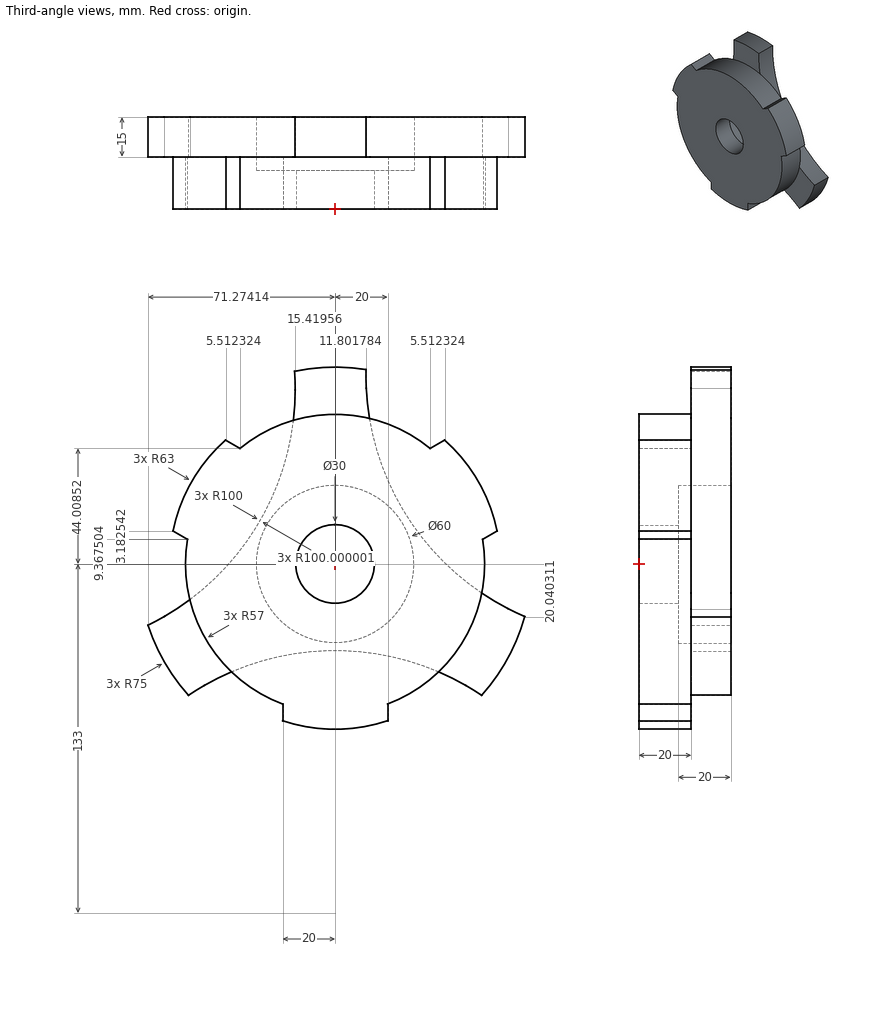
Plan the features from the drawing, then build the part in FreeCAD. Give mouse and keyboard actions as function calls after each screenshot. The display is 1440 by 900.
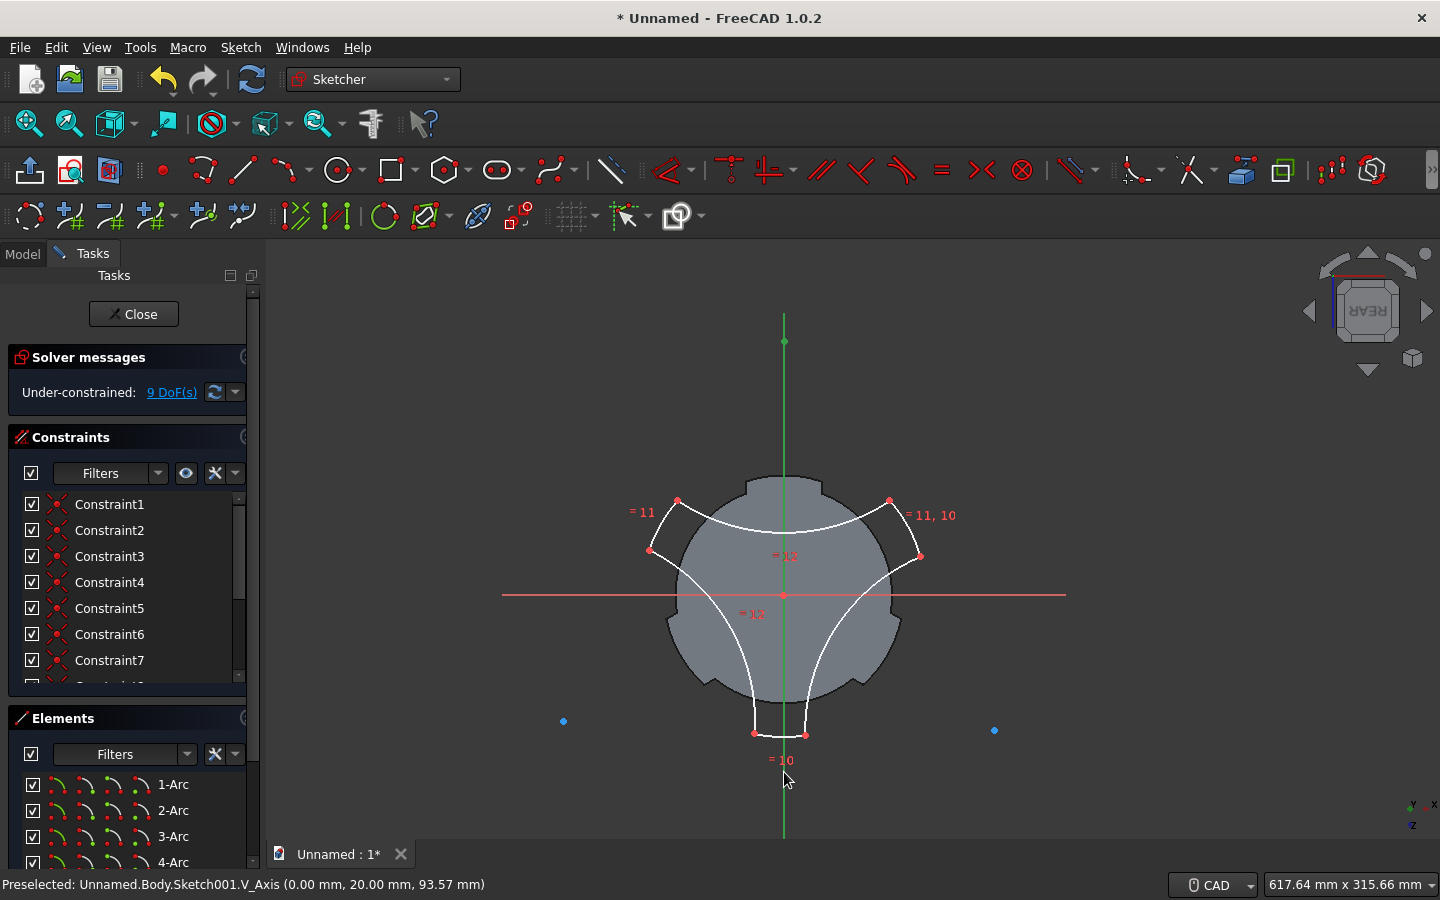
click(730, 170)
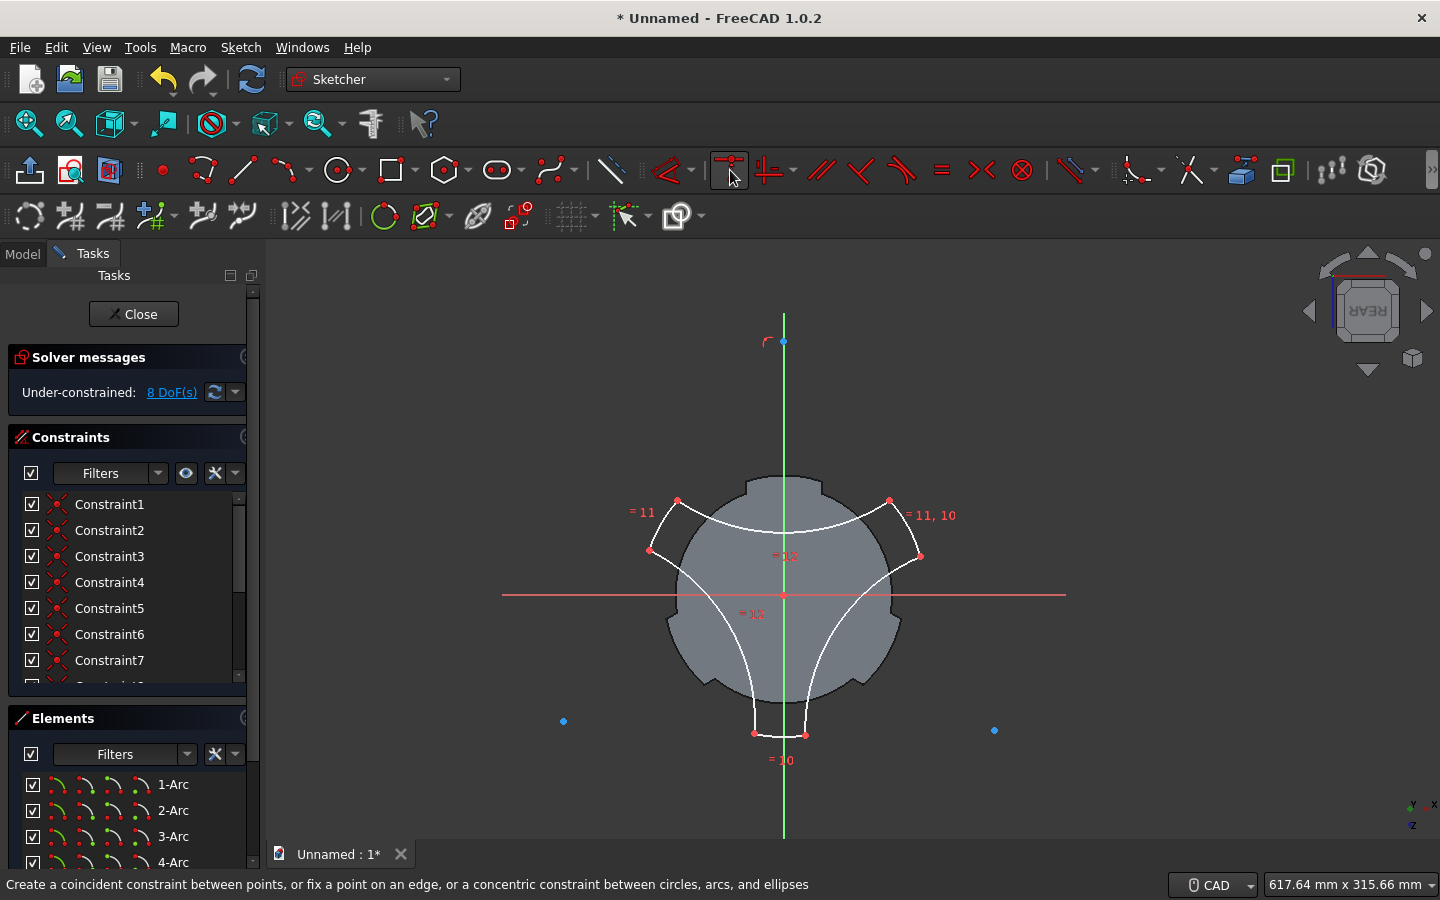
key(d)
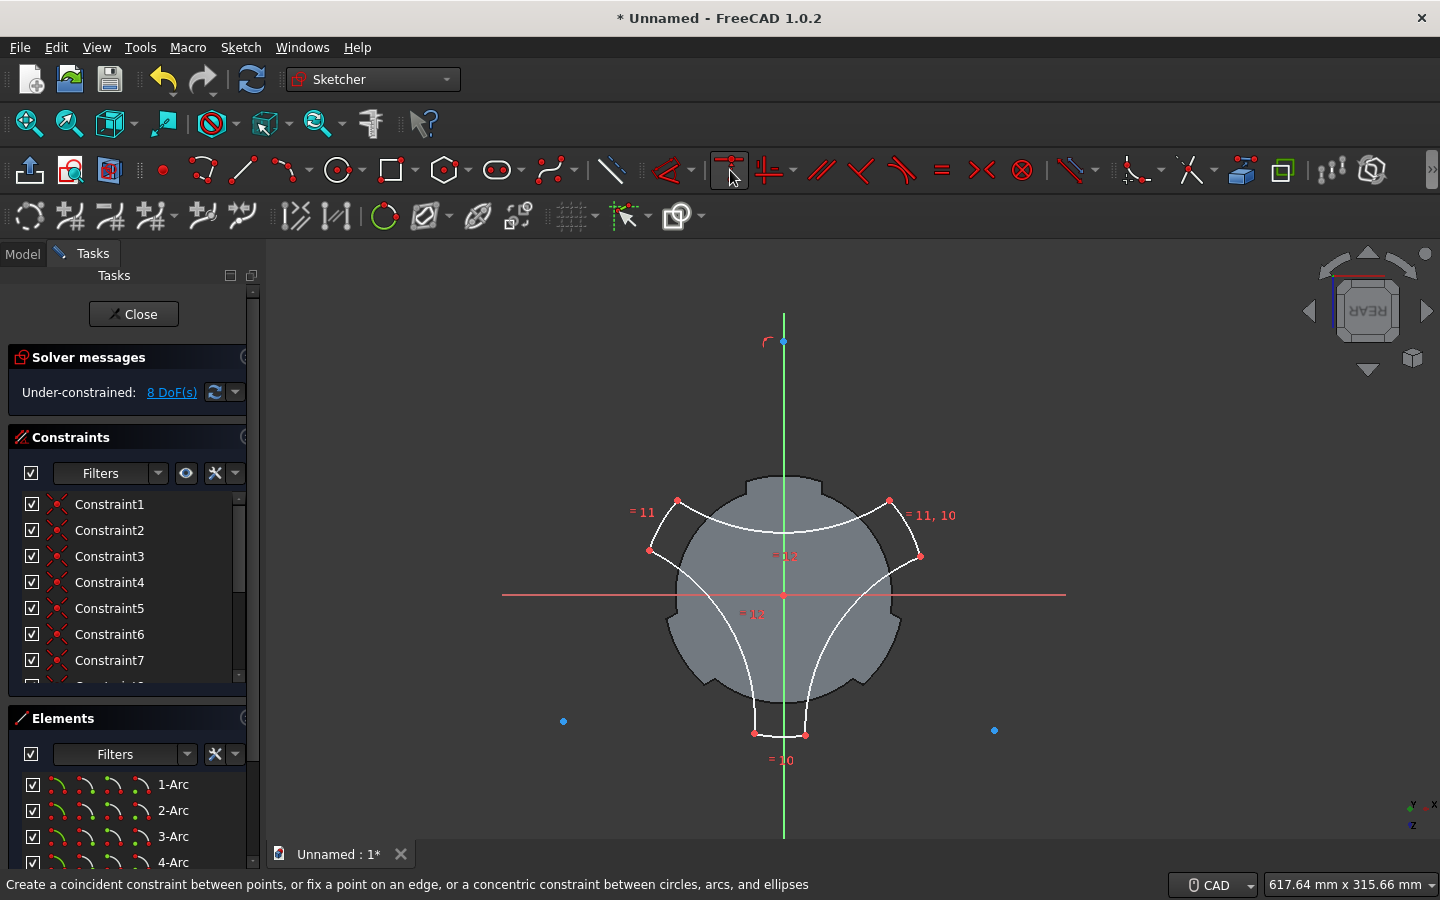
click(747, 667)
click(721, 563)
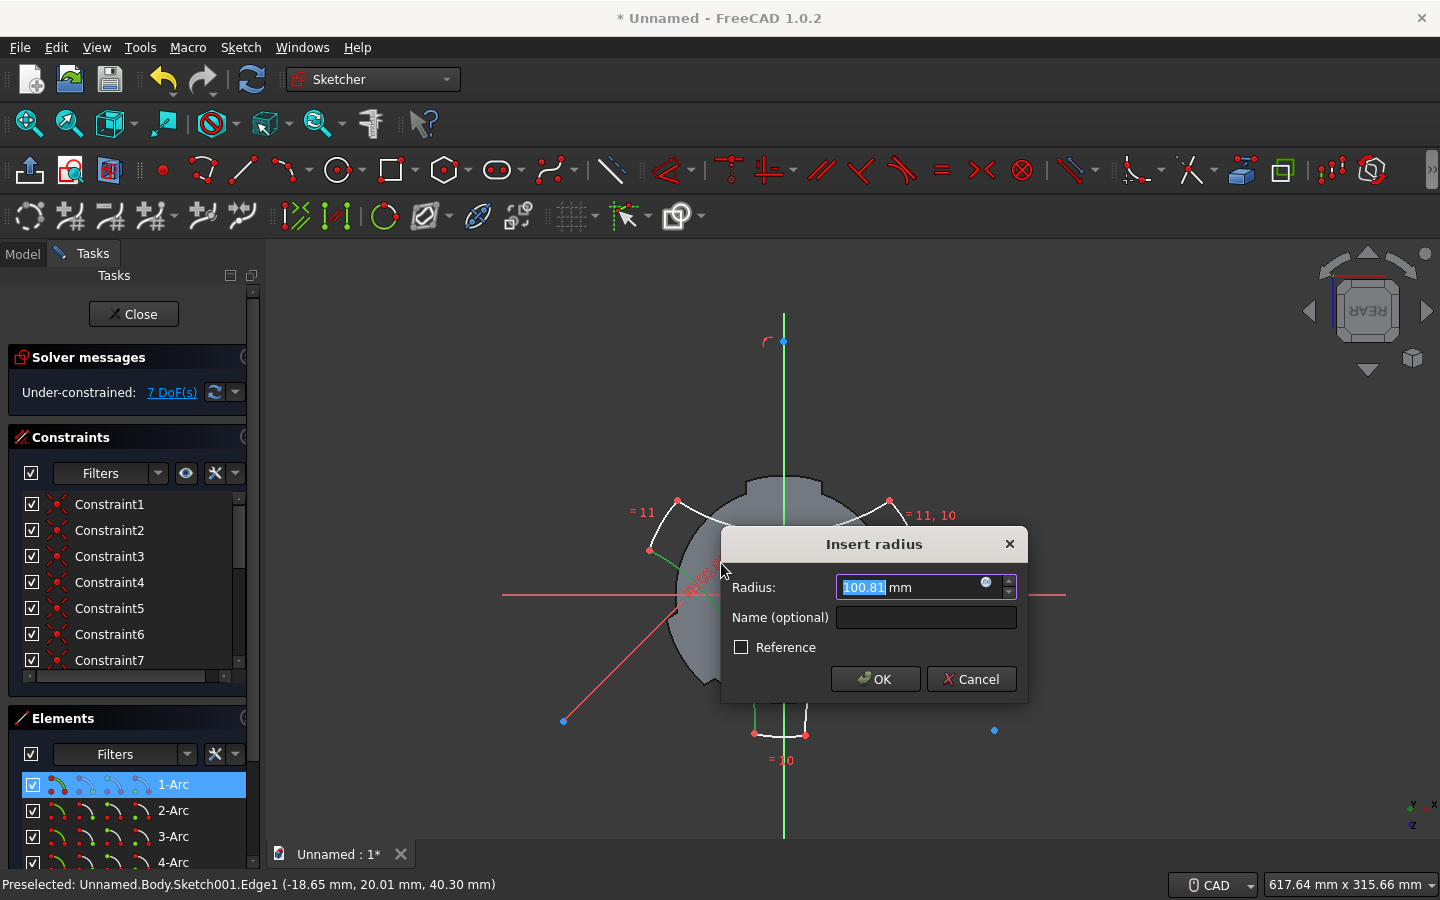
text(100.000001)
key(Return)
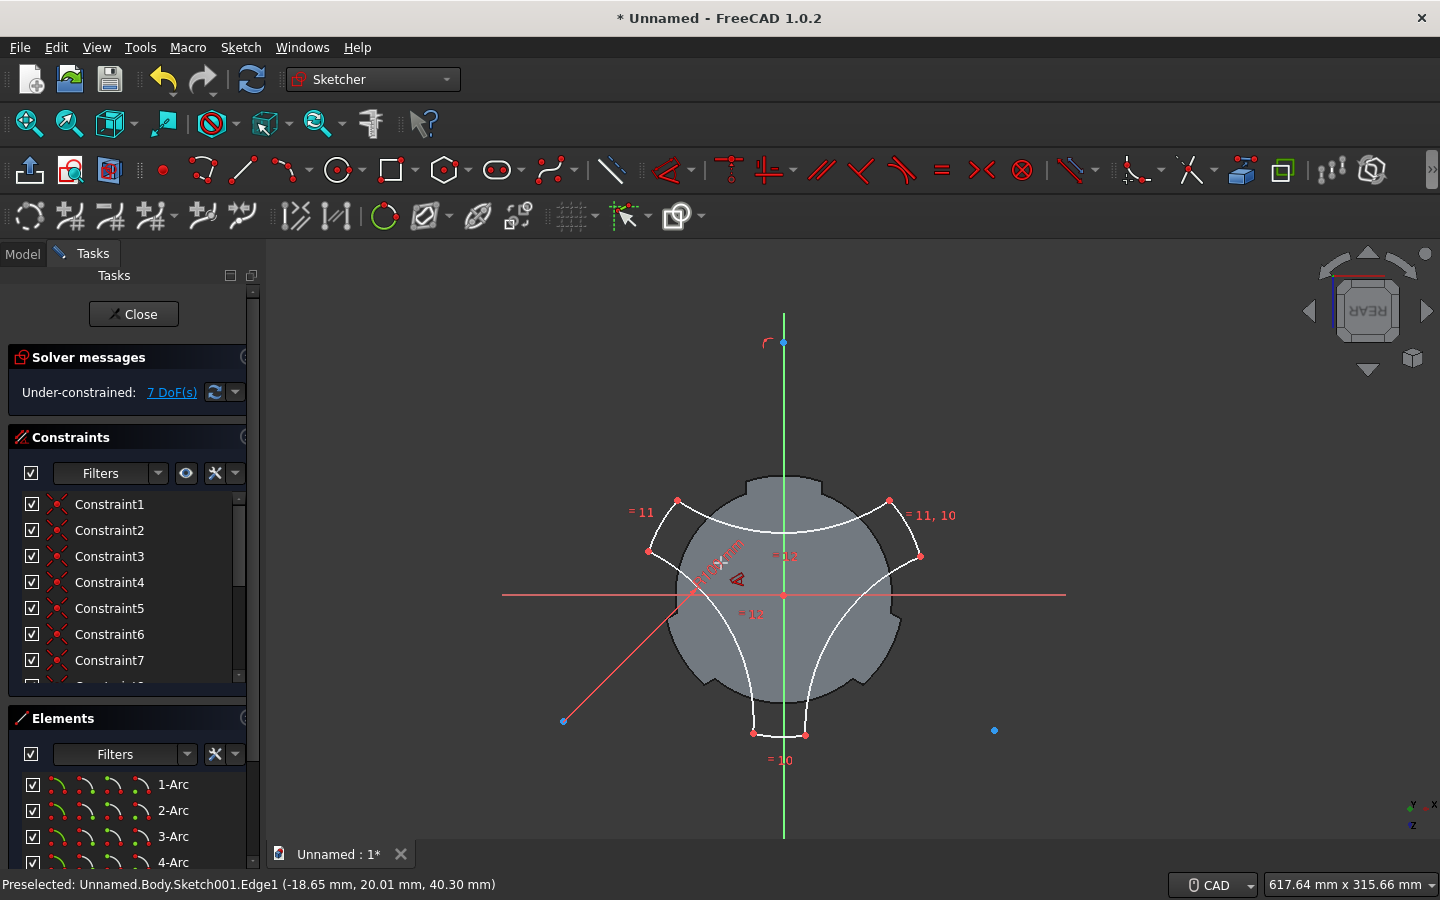
click(769, 736)
click(766, 768)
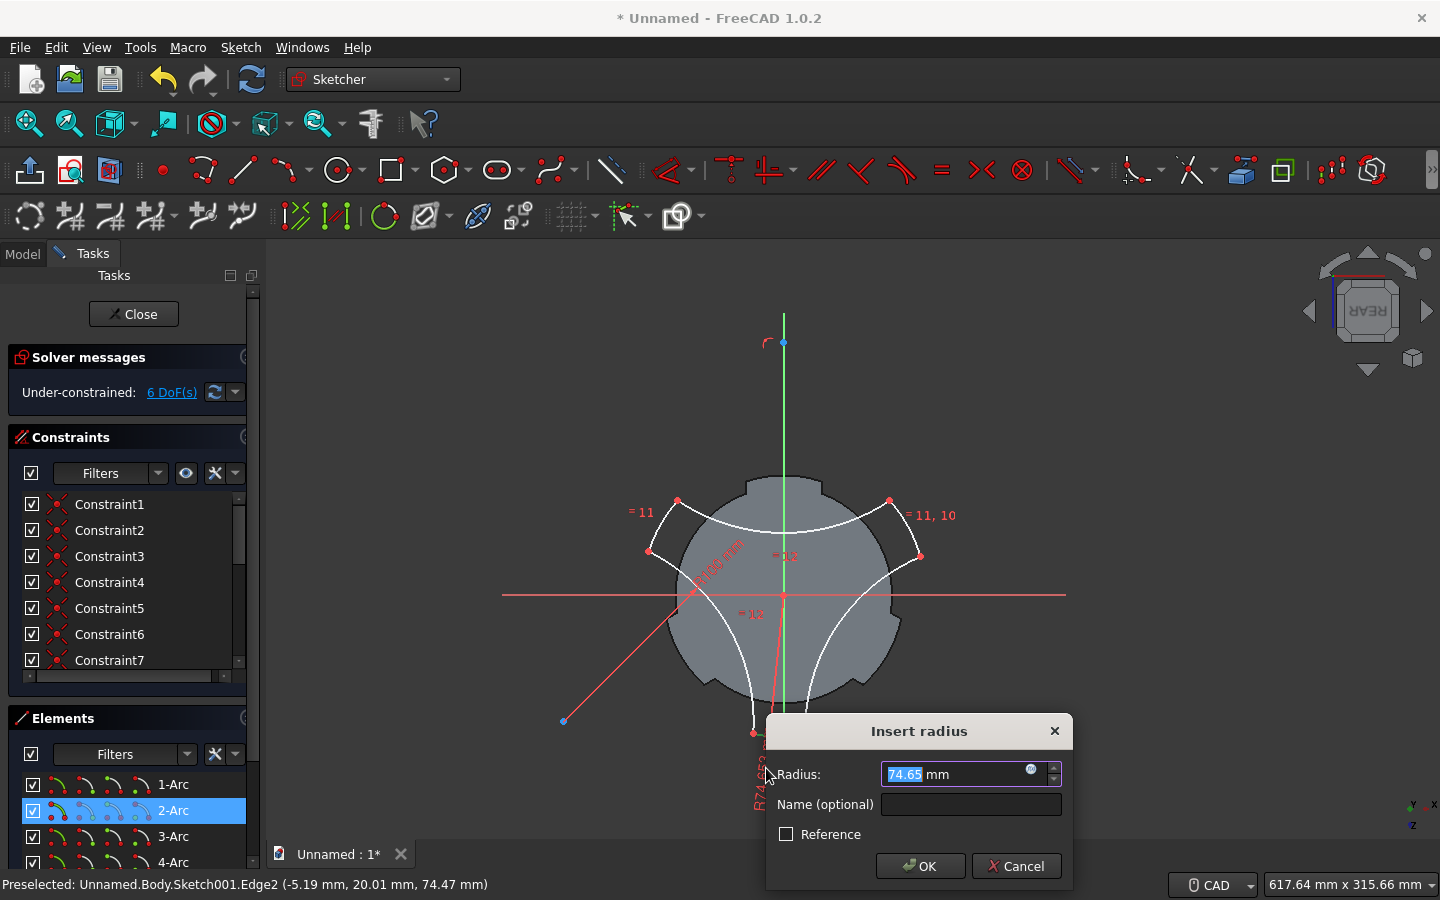
text(75)
key(Return)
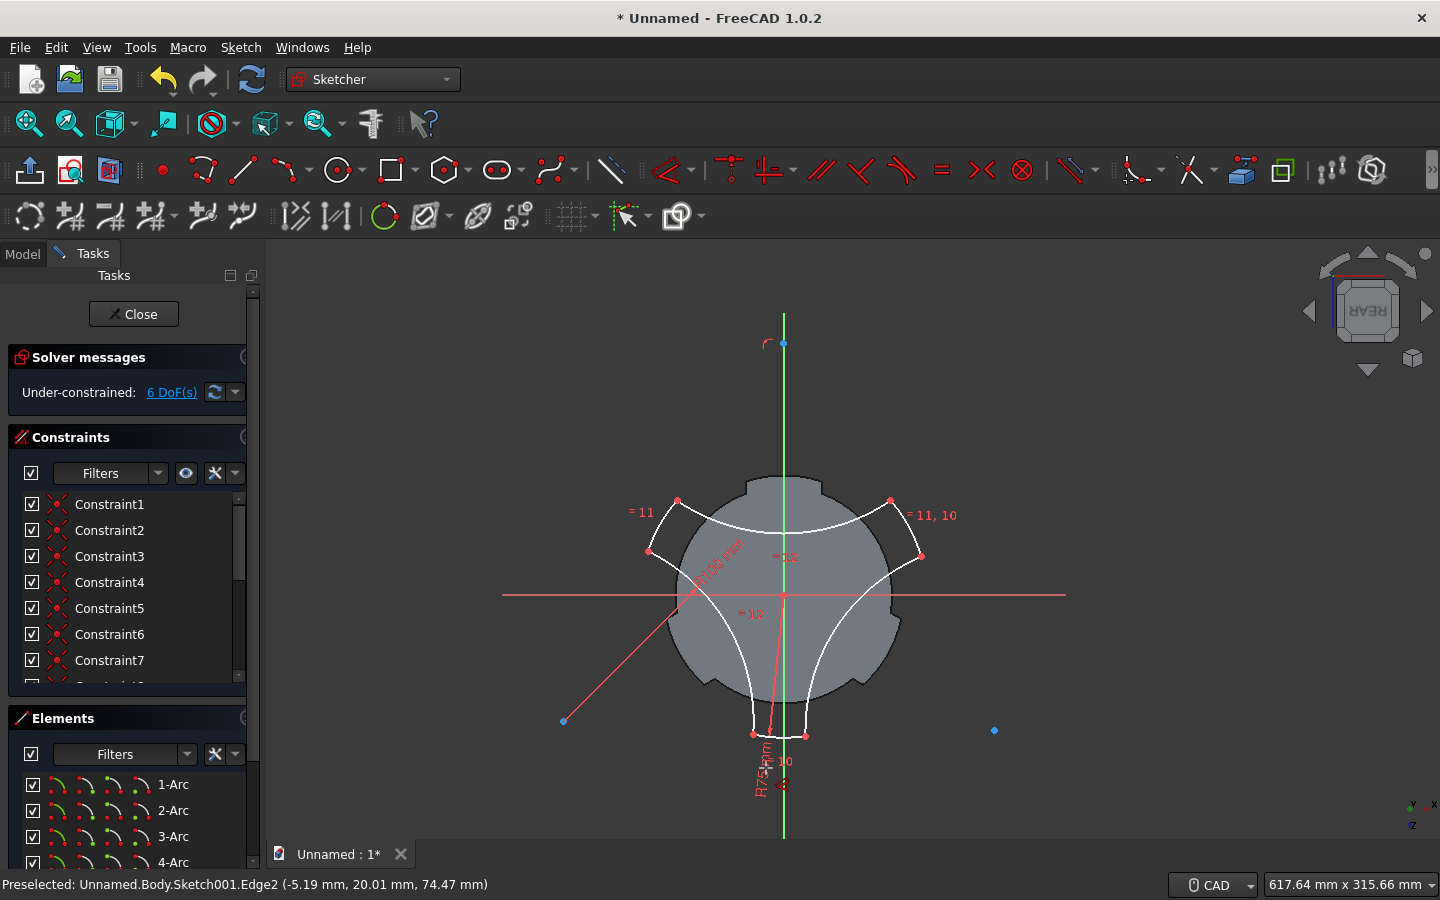
click(864, 594)
click(842, 571)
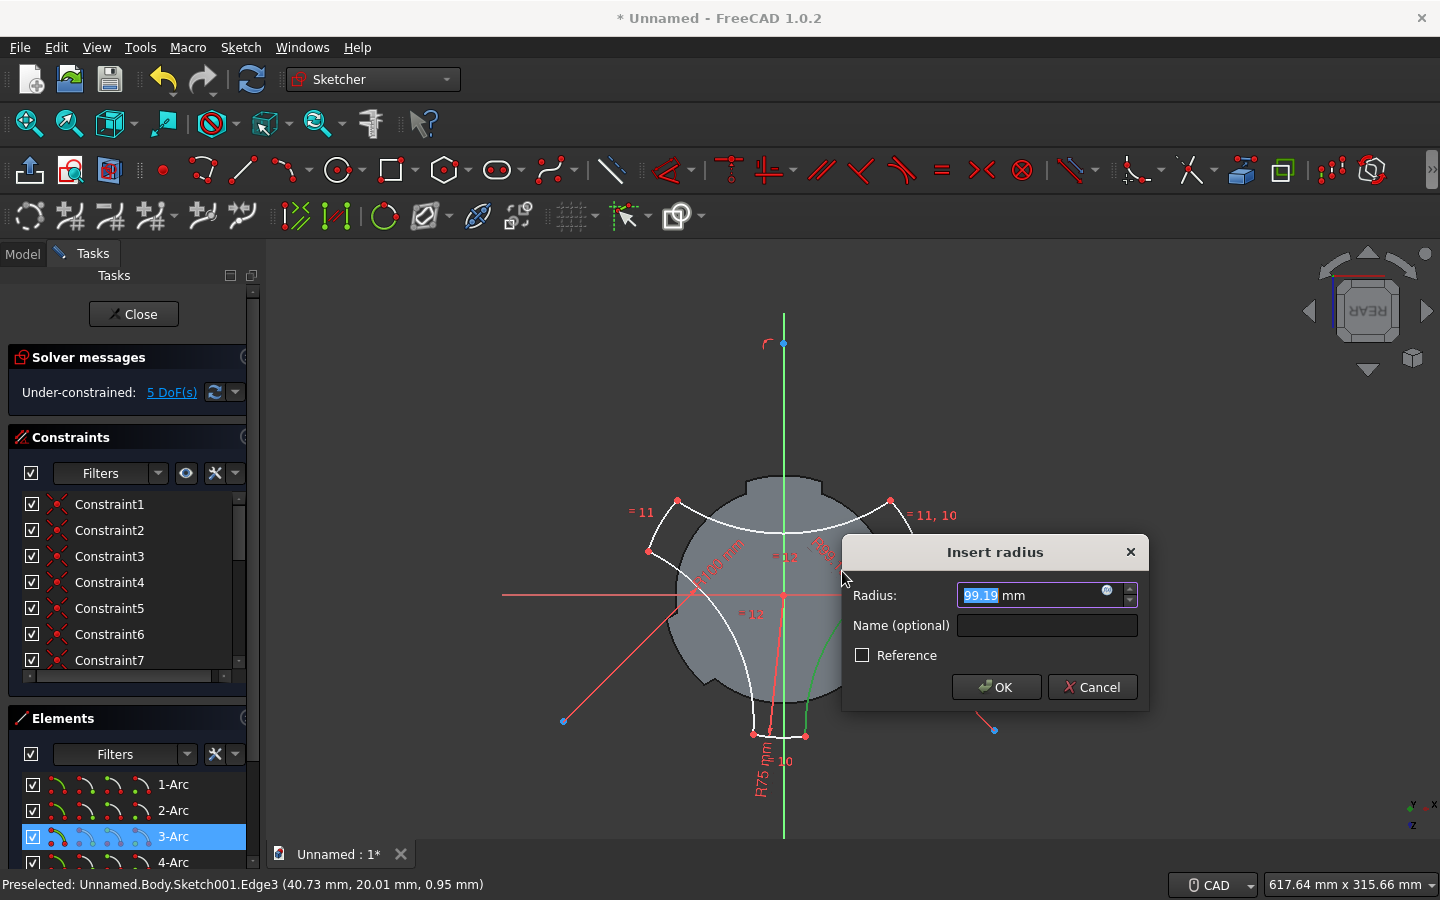
text(100)
key(Return)